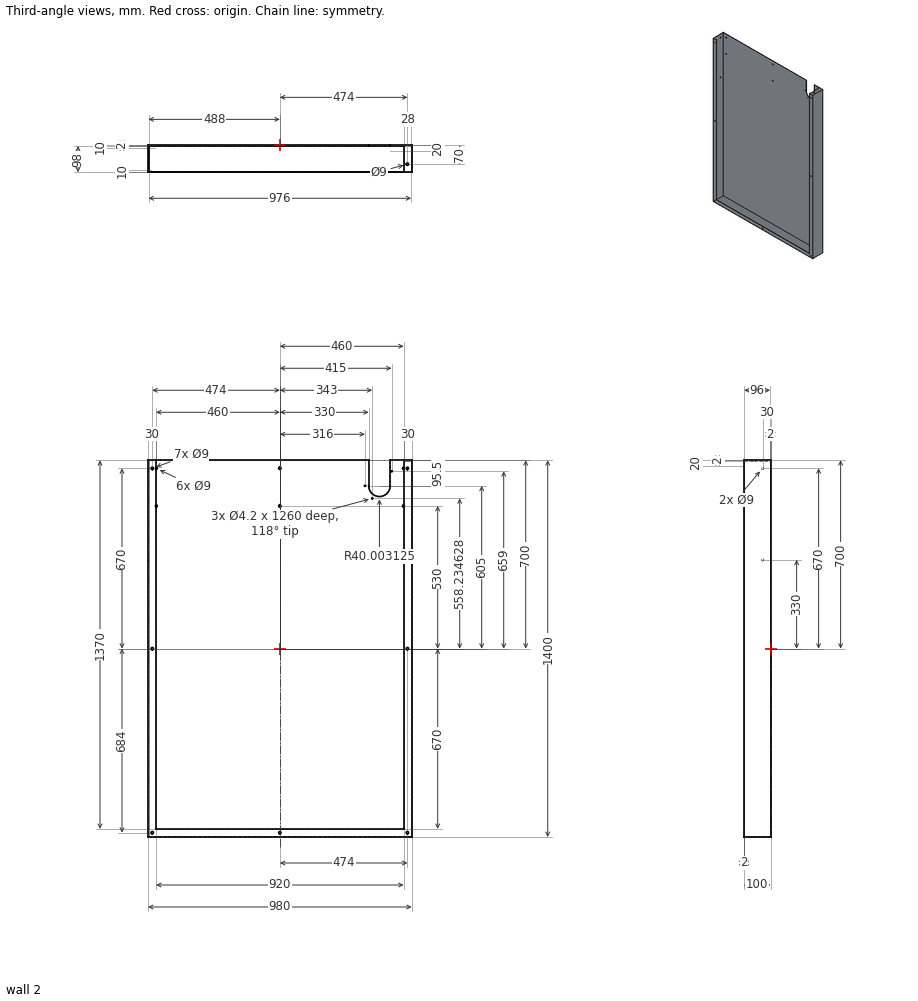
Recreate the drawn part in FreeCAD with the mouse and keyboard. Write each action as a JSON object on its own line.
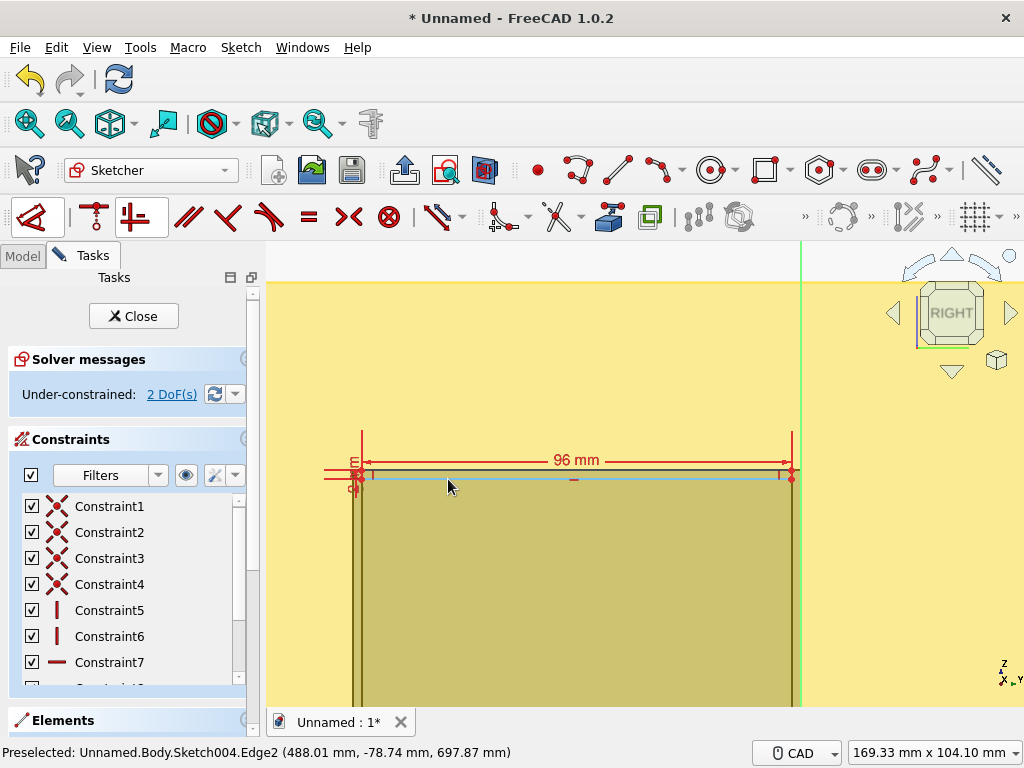
{"action": "scroll", "coordinate": [792, 479], "scroll_direction": "up", "scroll_amount": 8}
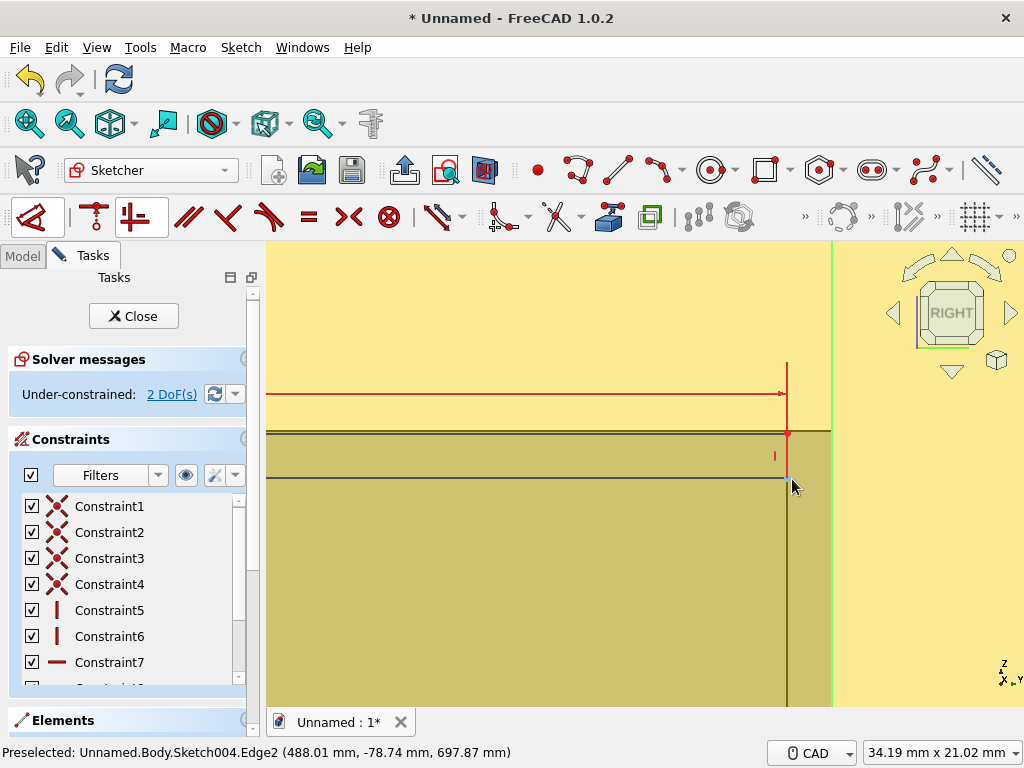
{"action": "left_click", "coordinate": [787, 478]}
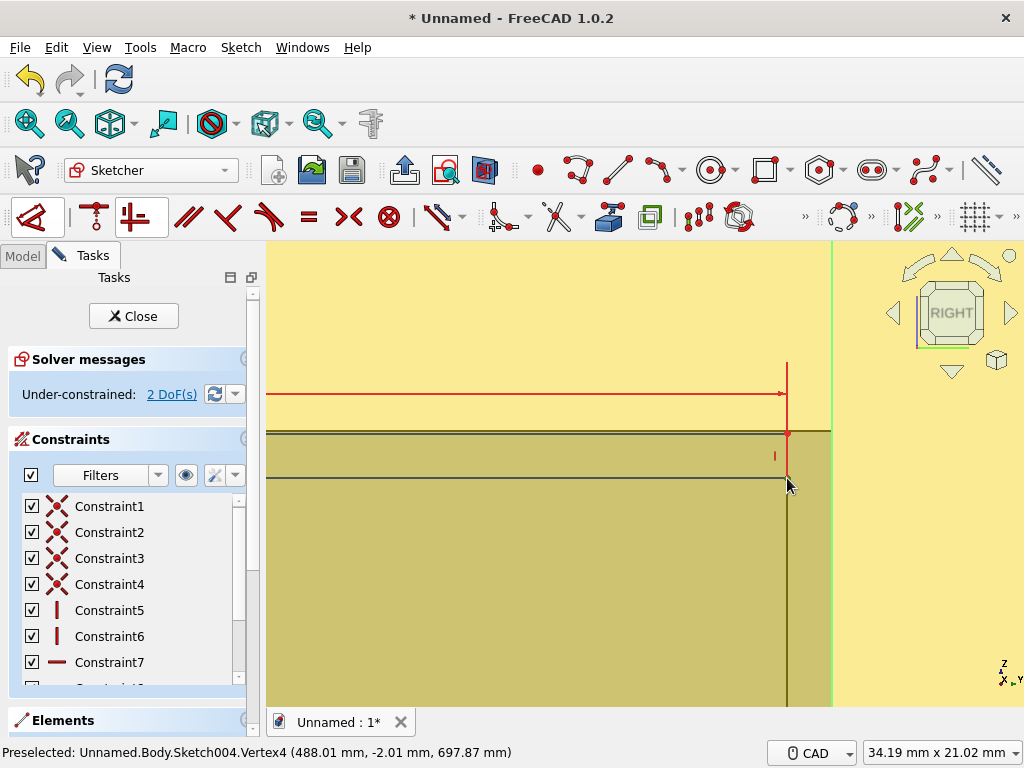
{"action": "key", "text": "l"}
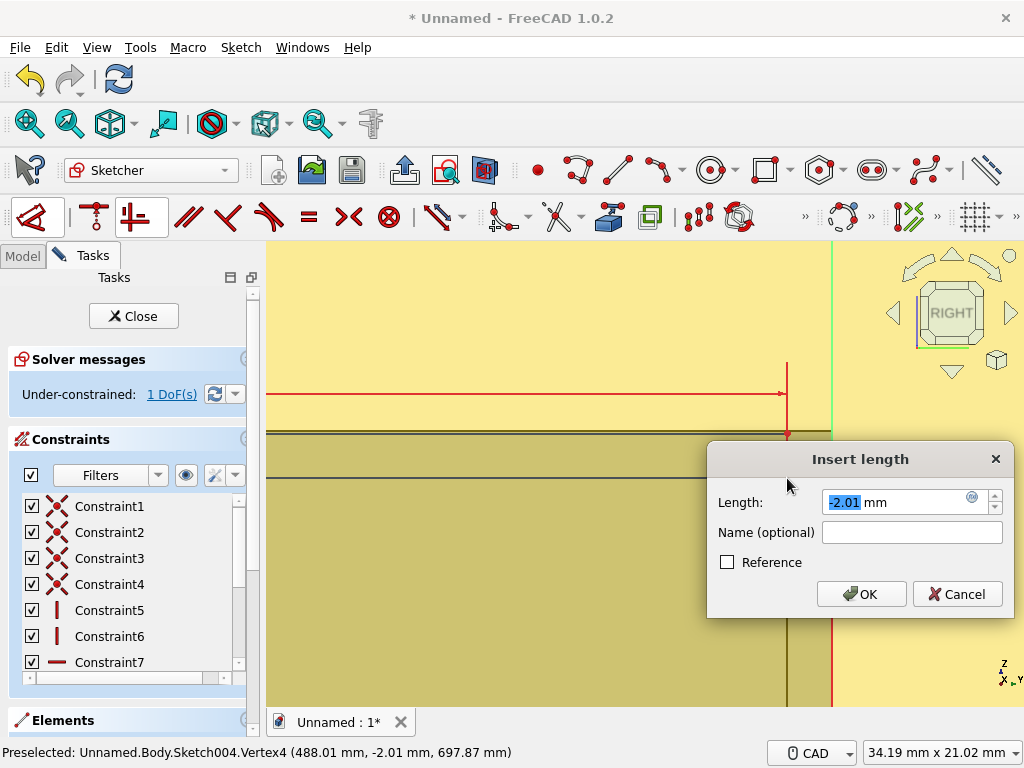
{"action": "type", "text": "-2"}
{"action": "key", "text": "Return"}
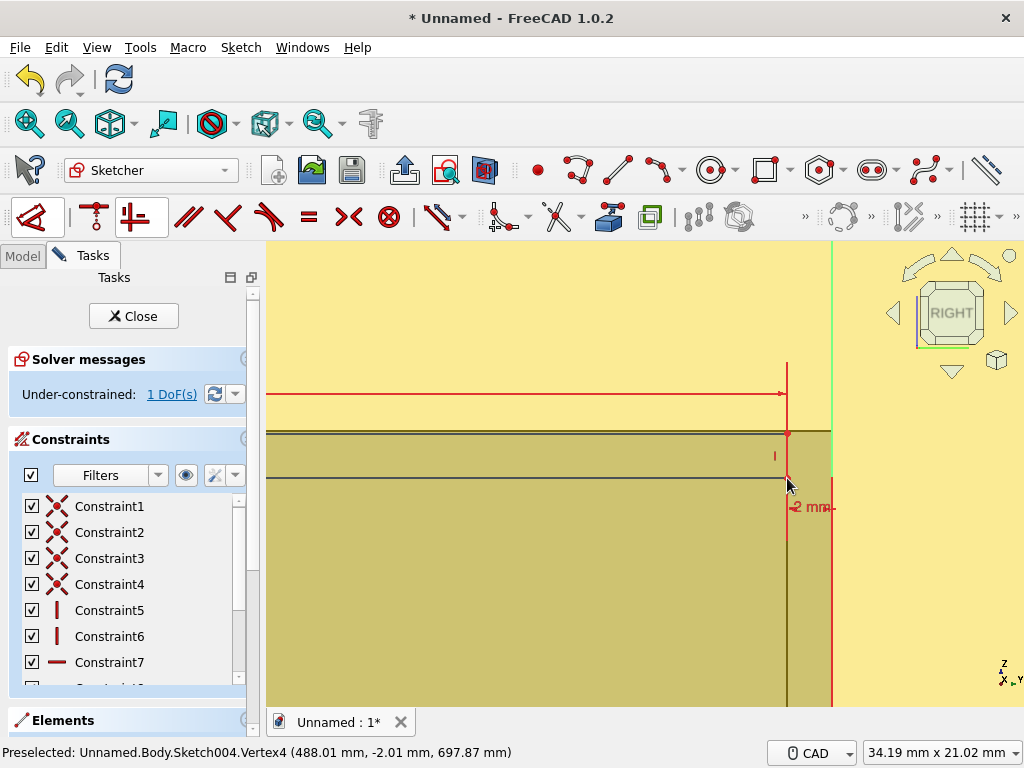
{"action": "scroll", "coordinate": [792, 479], "scroll_direction": "down", "scroll_amount": 8}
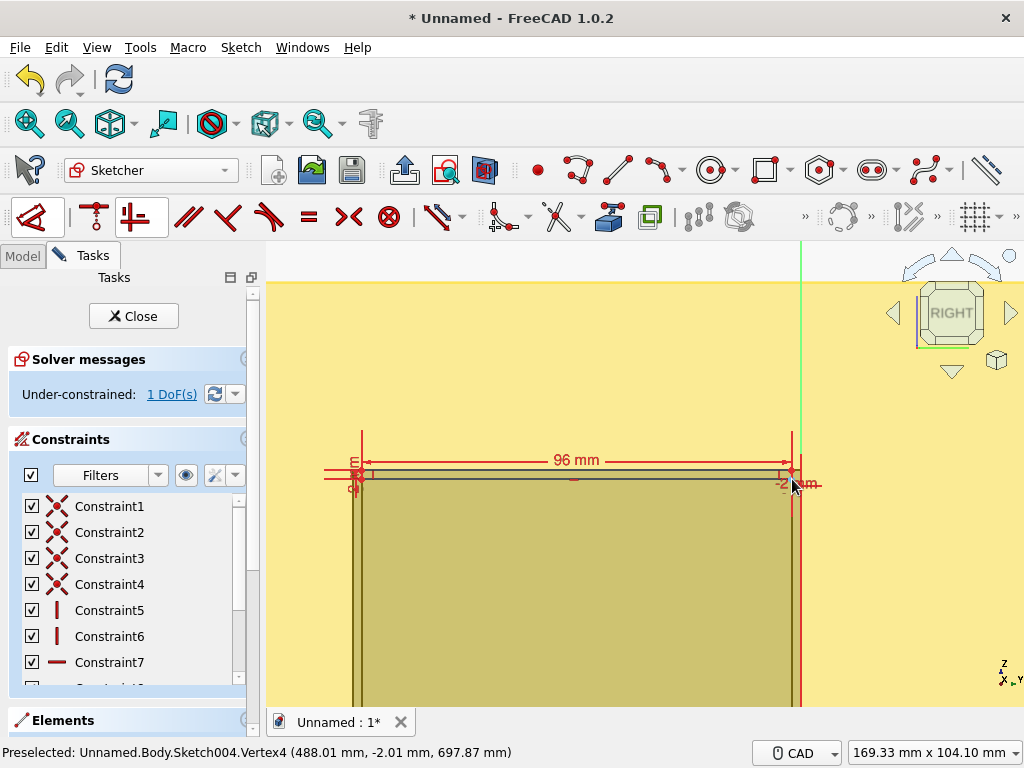
{"action": "scroll", "coordinate": [362, 470], "scroll_direction": "up", "scroll_amount": 2}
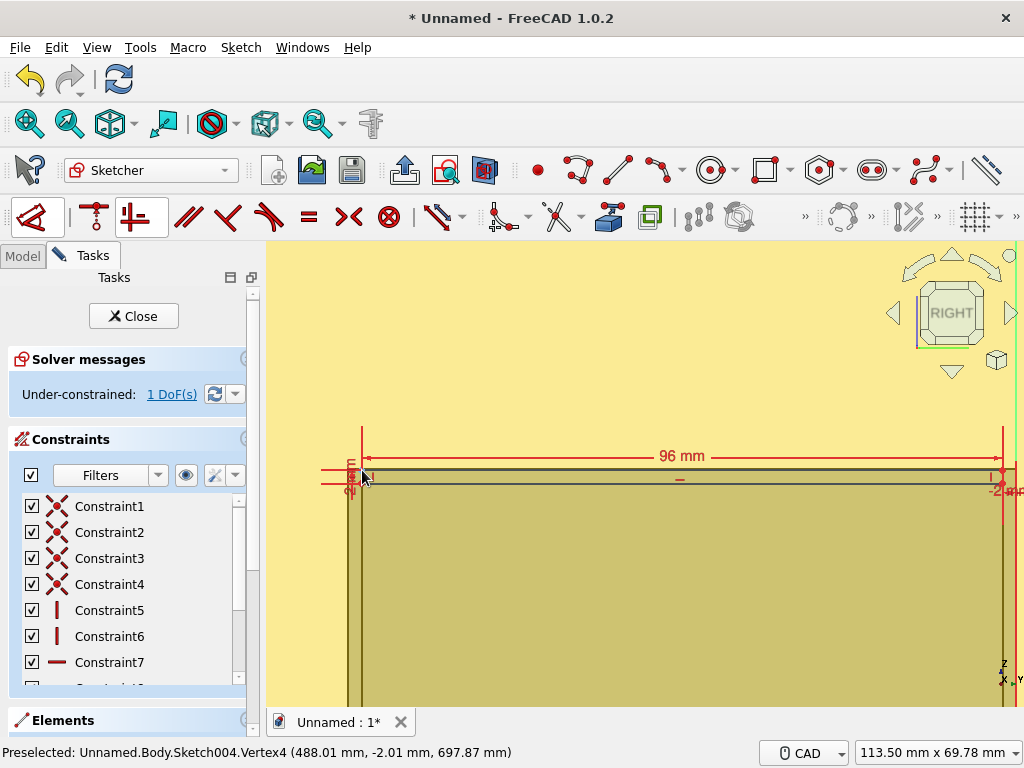
{"action": "left_click", "coordinate": [362, 470]}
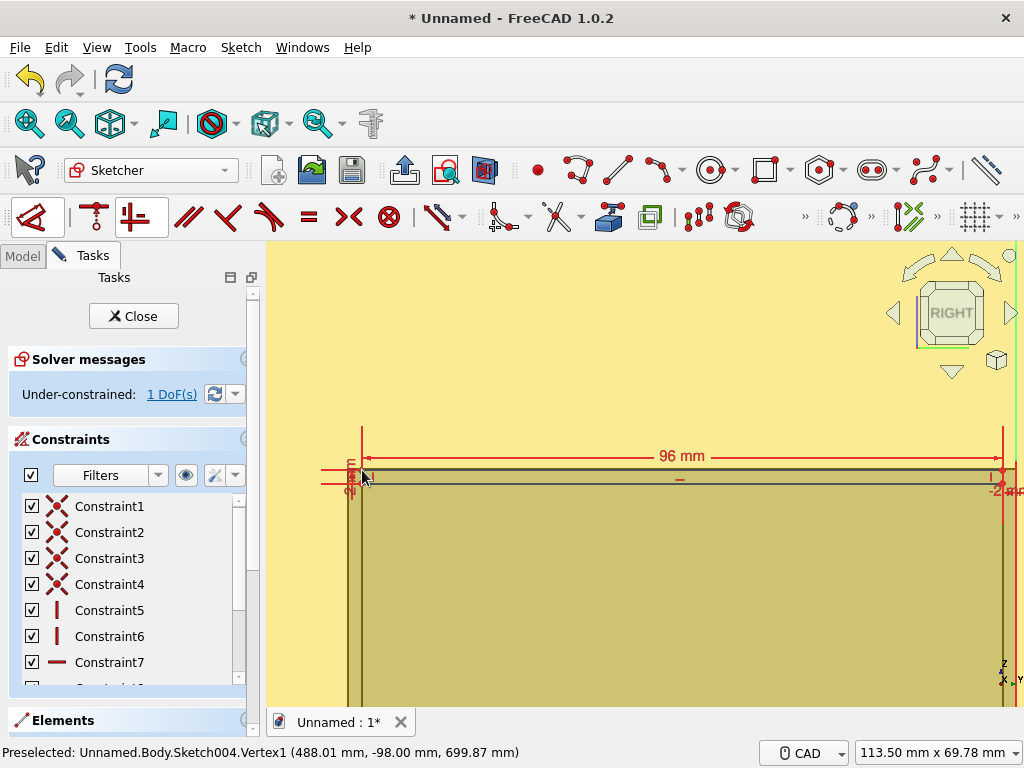
{"action": "left_click", "coordinate": [58, 218]}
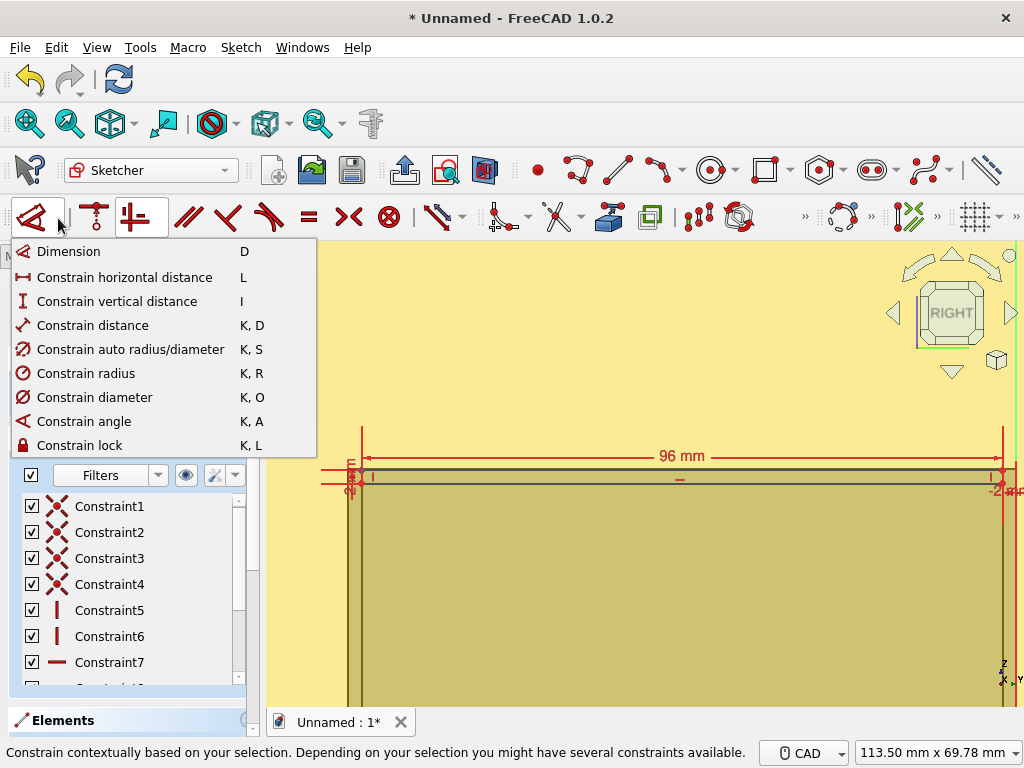
{"action": "left_click", "coordinate": [164, 301]}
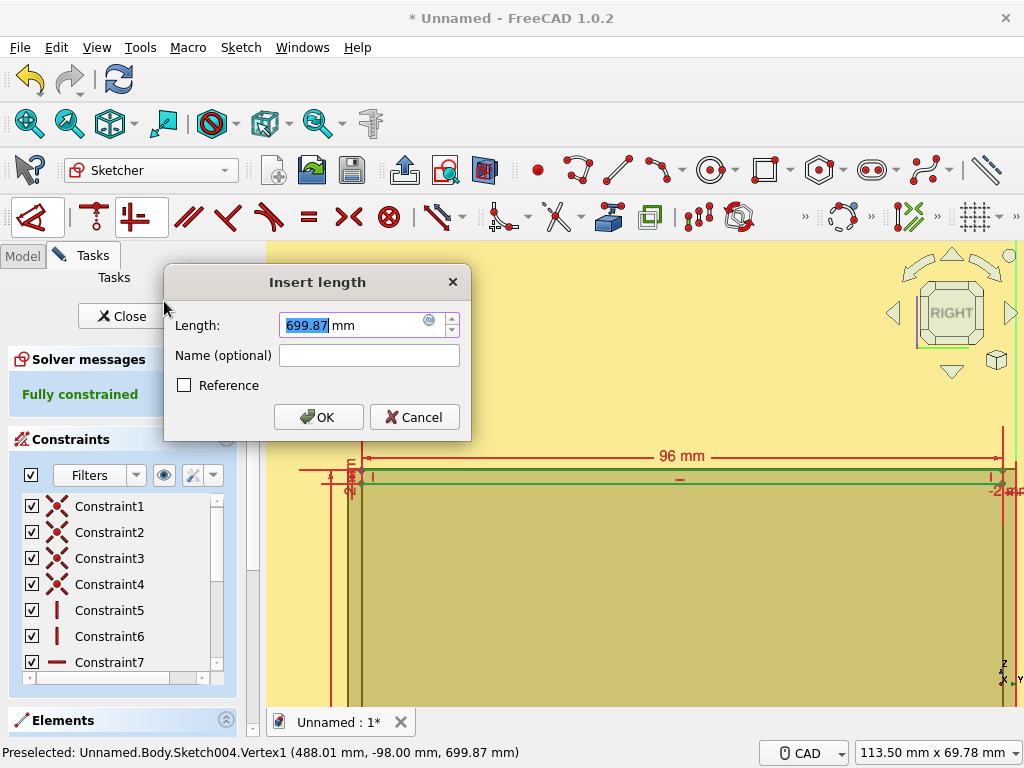
{"action": "type", "text": "700"}
{"action": "key", "text": "Return"}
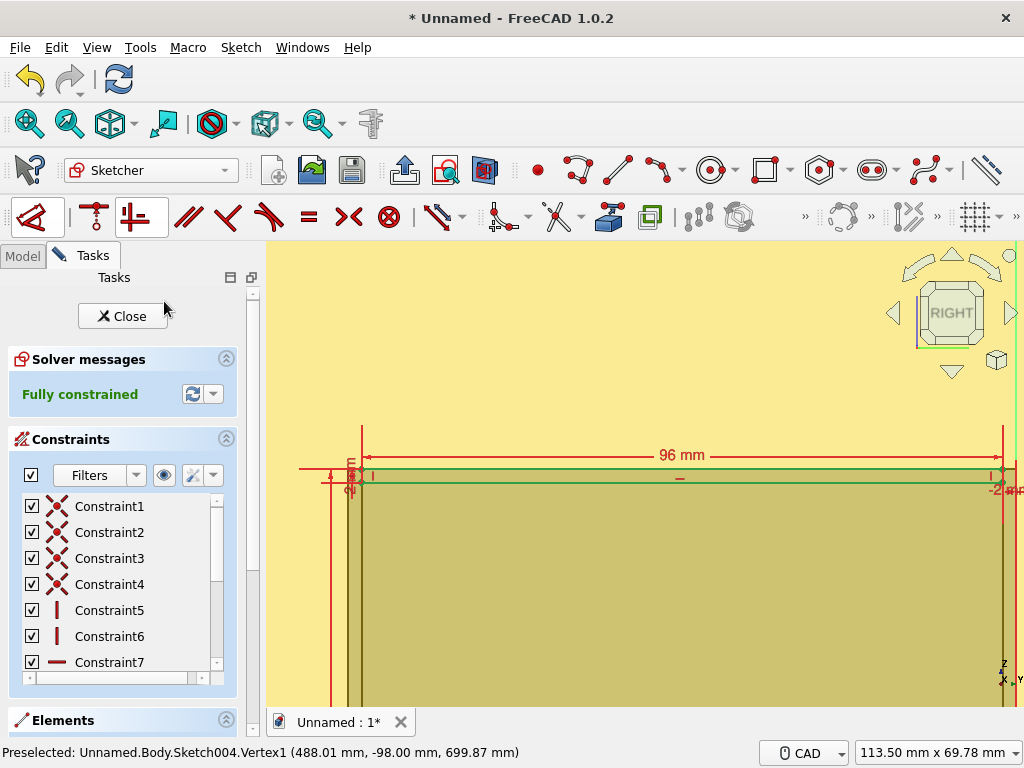
{"action": "left_click", "coordinate": [123, 316]}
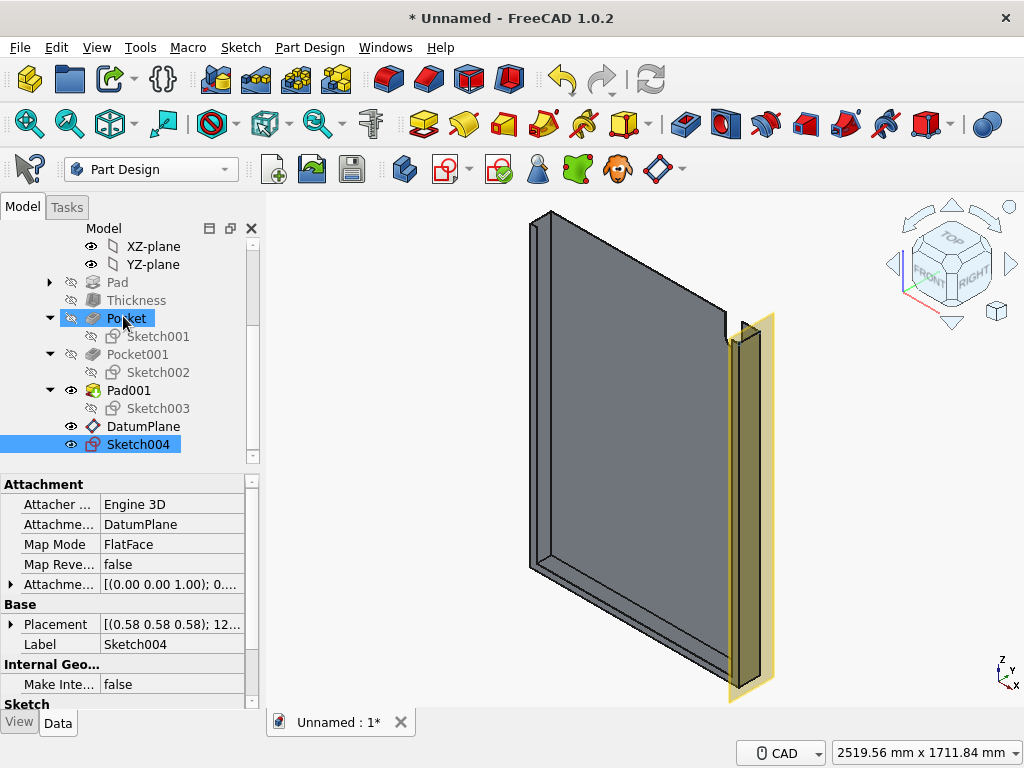
{"action": "left_click", "coordinate": [424, 124]}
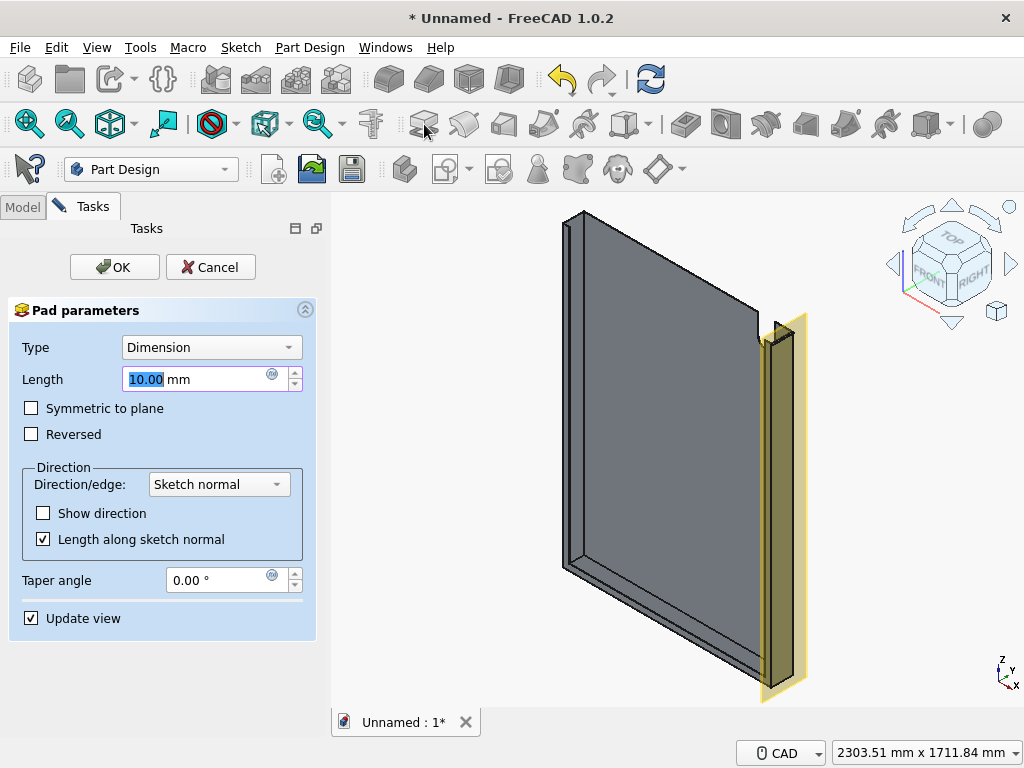
{"action": "type", "text": "28"}
{"action": "key", "text": "Tab"}